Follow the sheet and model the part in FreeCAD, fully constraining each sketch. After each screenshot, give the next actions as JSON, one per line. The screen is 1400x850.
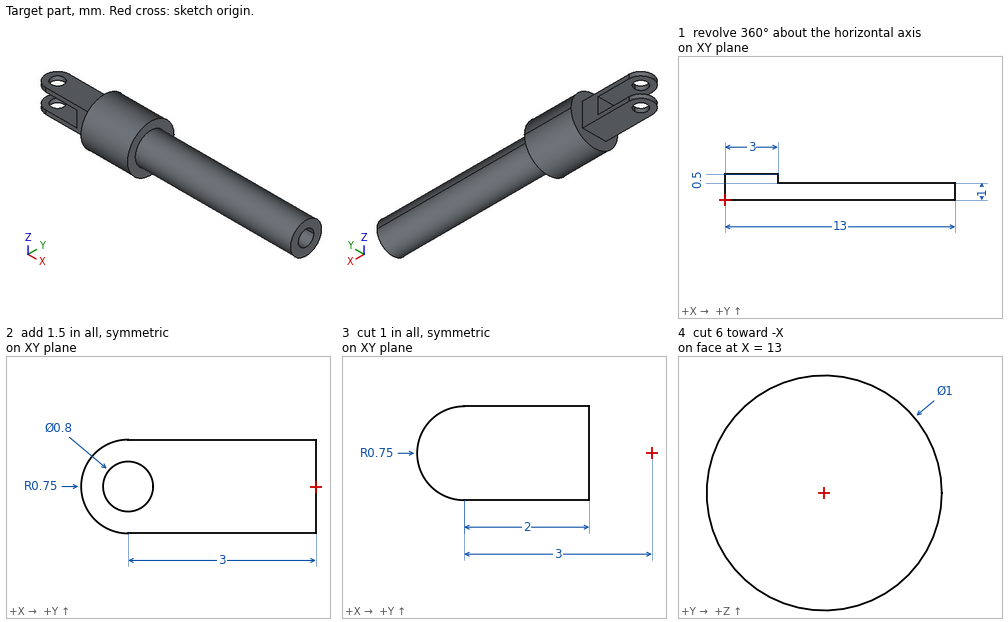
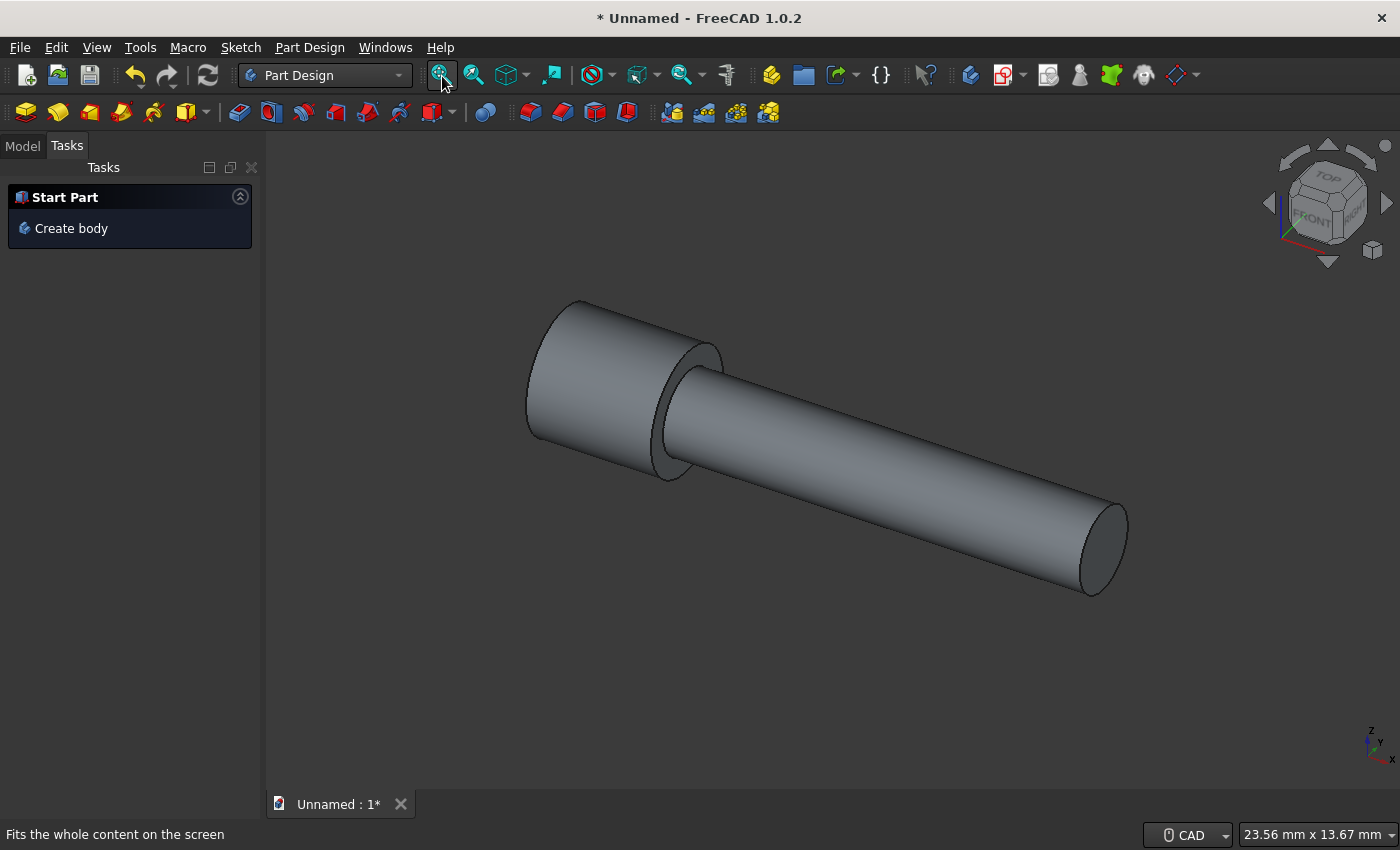
{"action": "left_click", "coordinate": [1004, 76]}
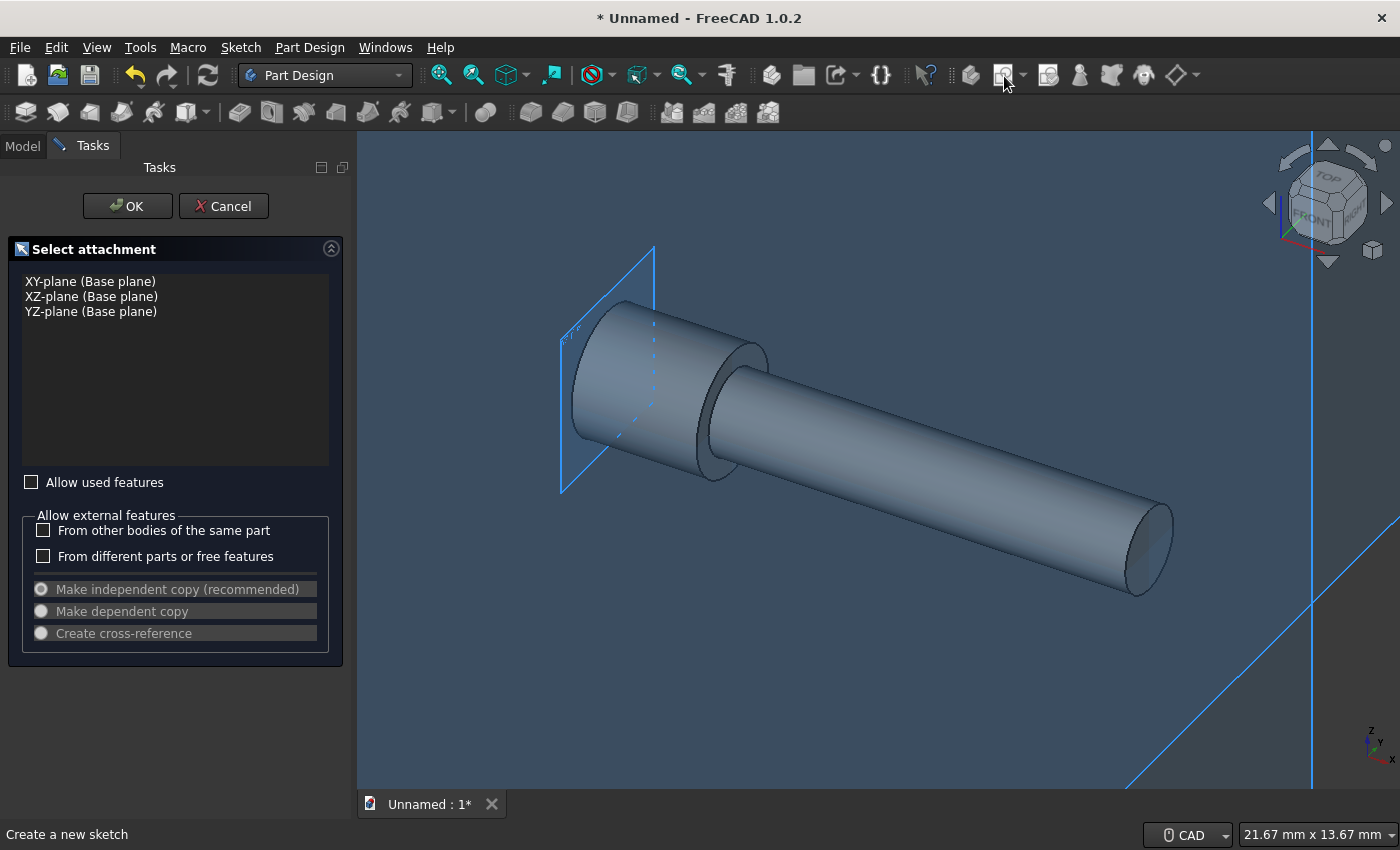
{"action": "left_click", "coordinate": [82, 282]}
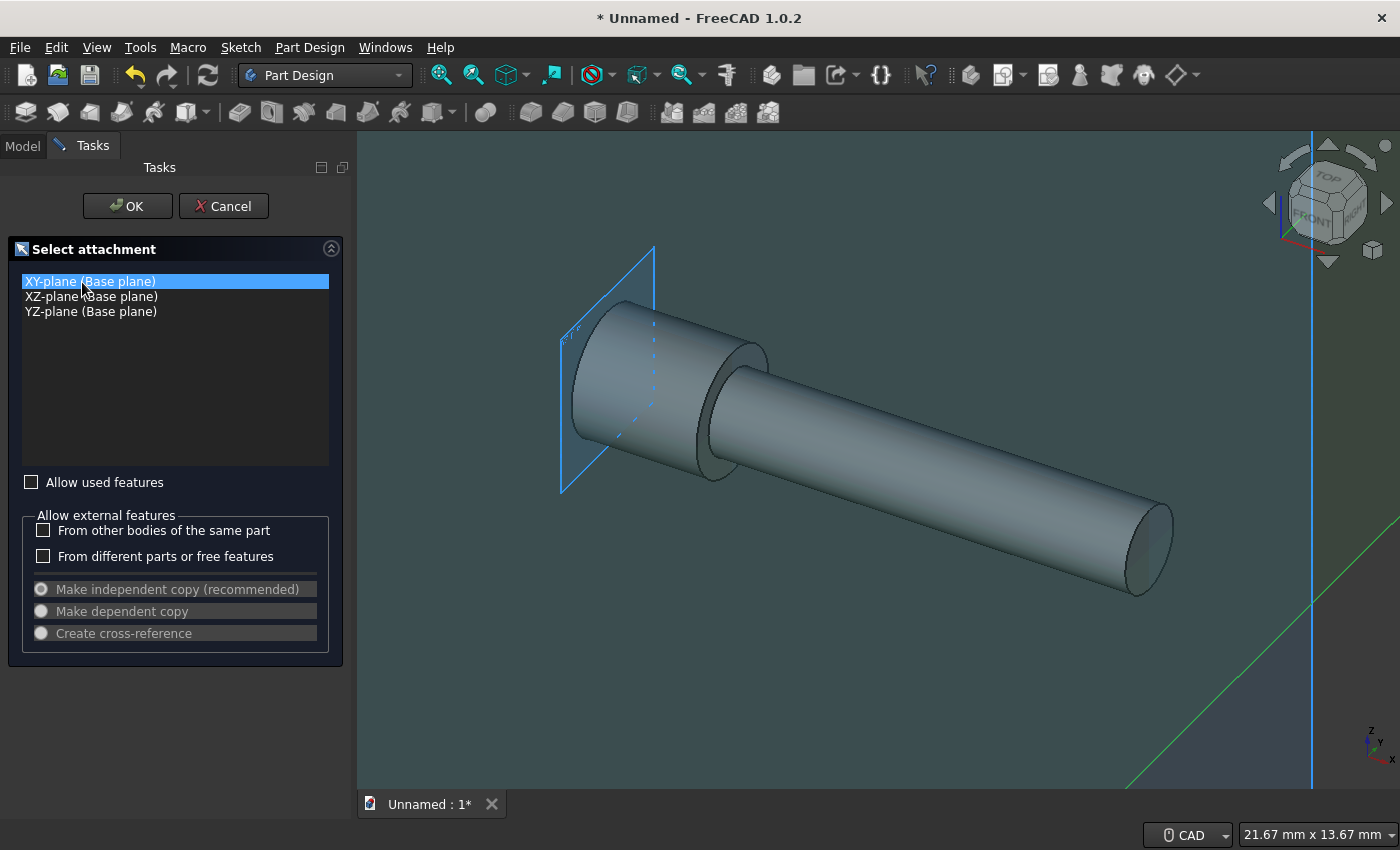
{"action": "left_click", "coordinate": [128, 206]}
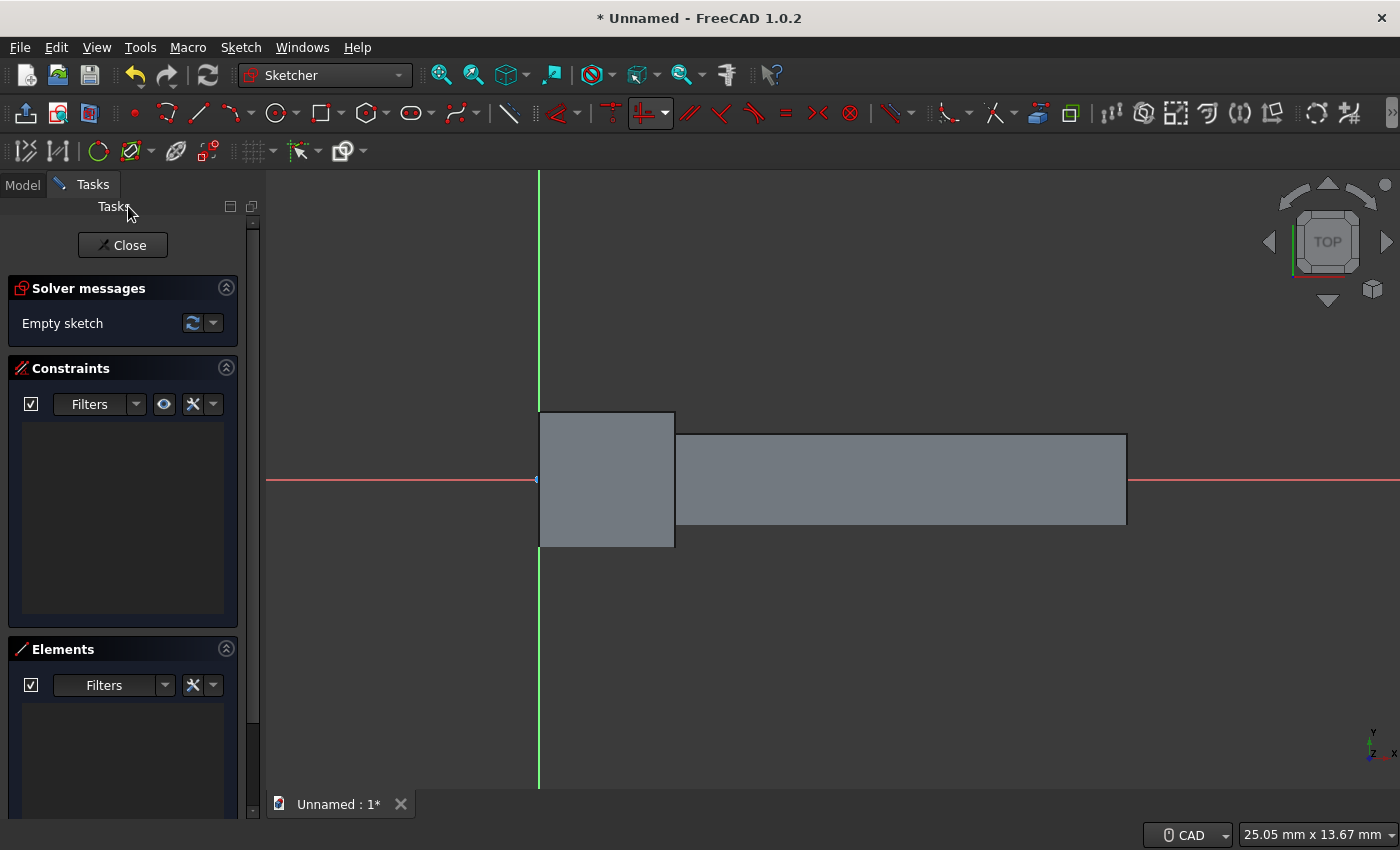
{"action": "key", "text": "q s"}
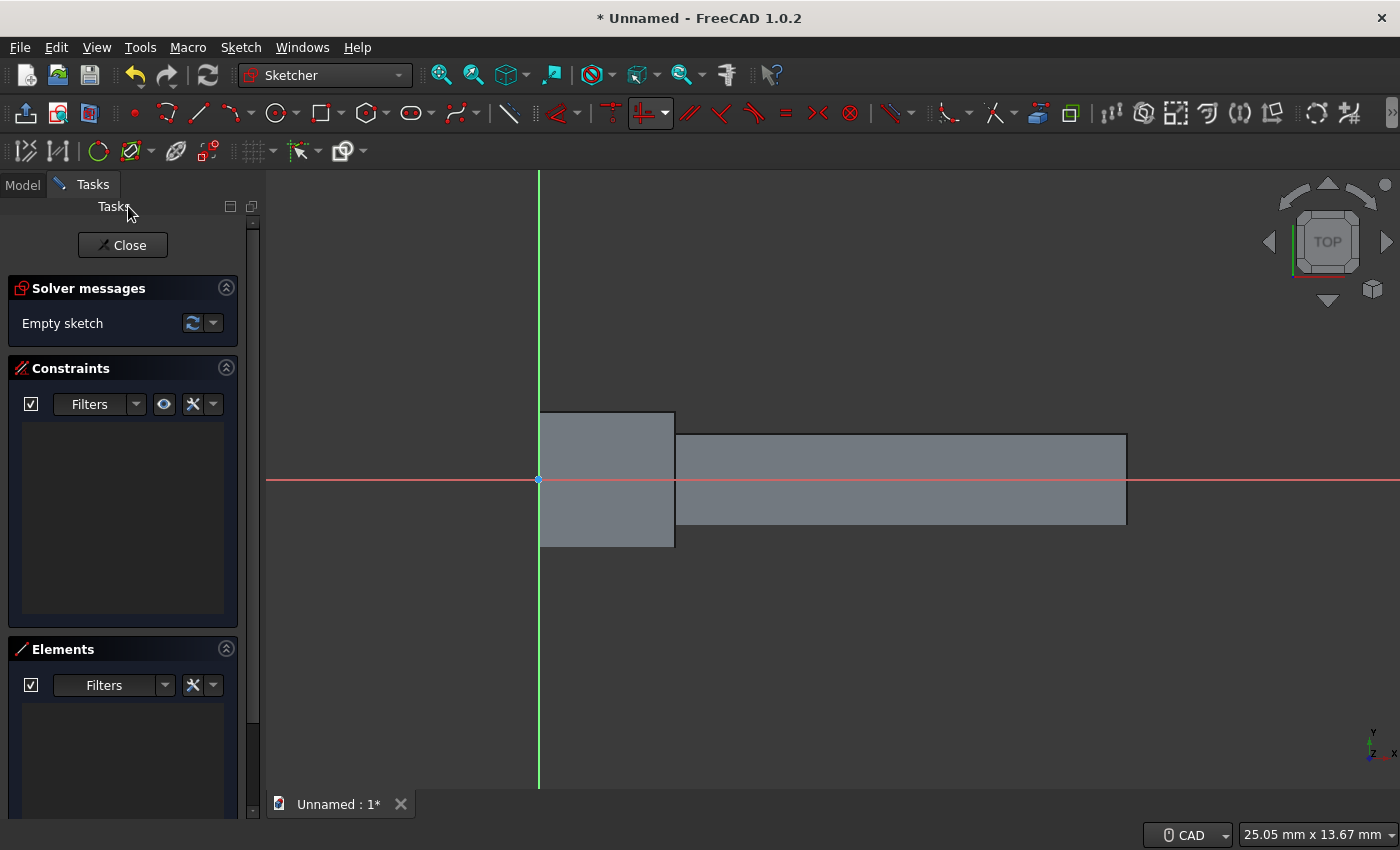
{"action": "scroll", "coordinate": [352, 480], "scroll_direction": "up", "scroll_amount": 7}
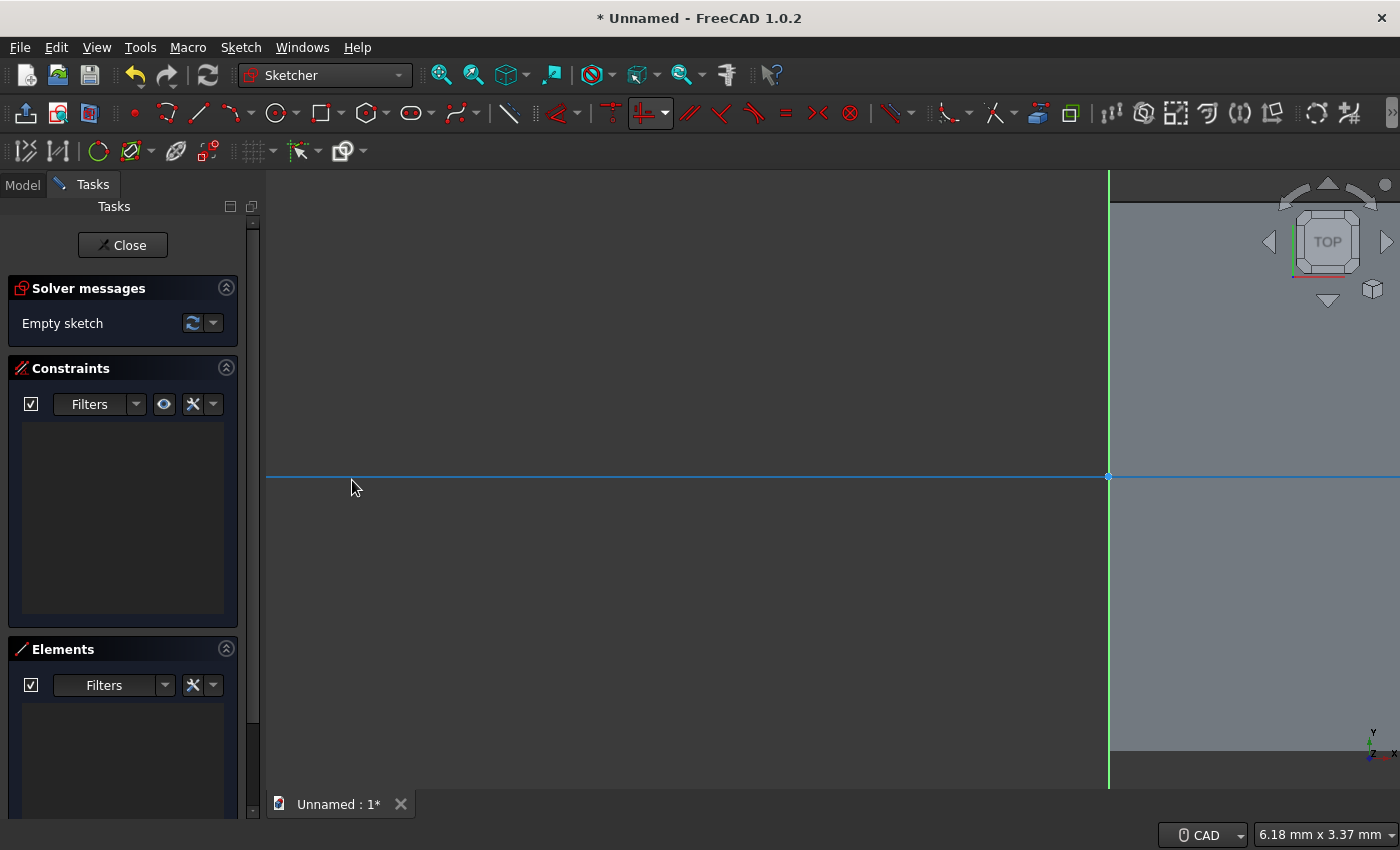
{"action": "left_click", "coordinate": [168, 114]}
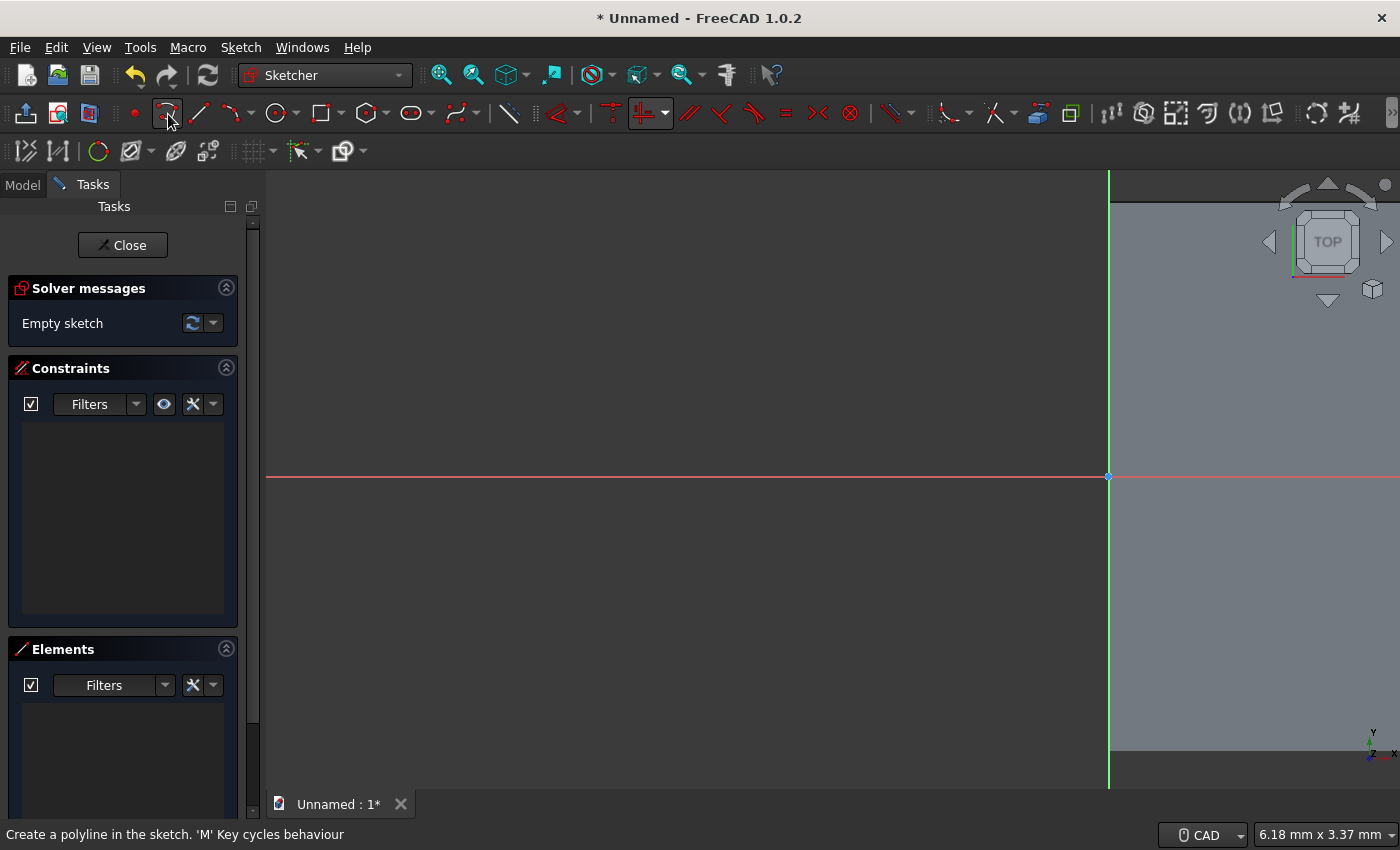
{"action": "left_click", "coordinate": [558, 615]}
{"action": "left_click", "coordinate": [1109, 615]}
{"action": "left_click", "coordinate": [1100, 339]}
{"action": "left_click", "coordinate": [558, 339]}
{"action": "right_click", "coordinate": [558, 339]}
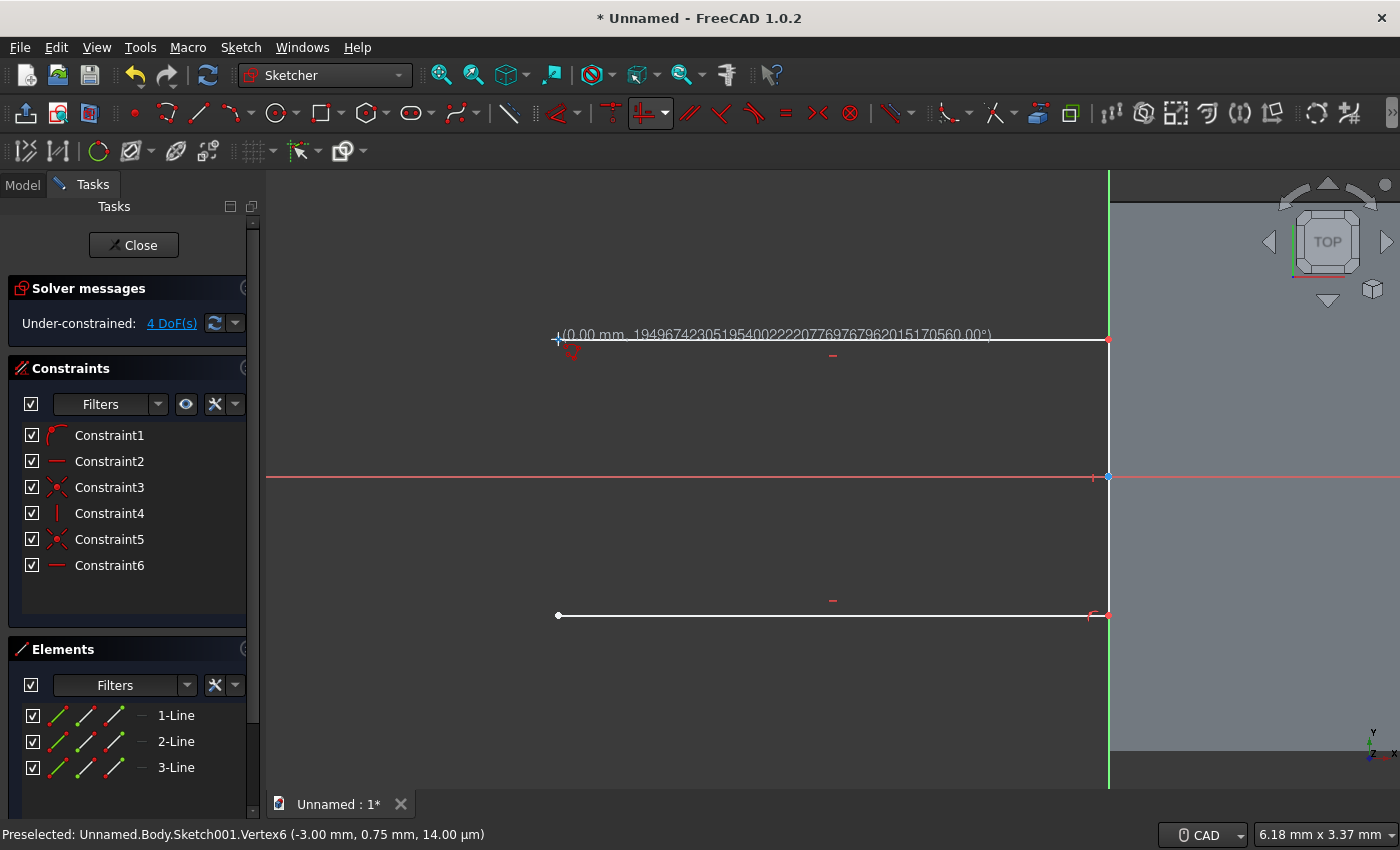
{"action": "left_click", "coordinate": [232, 114]}